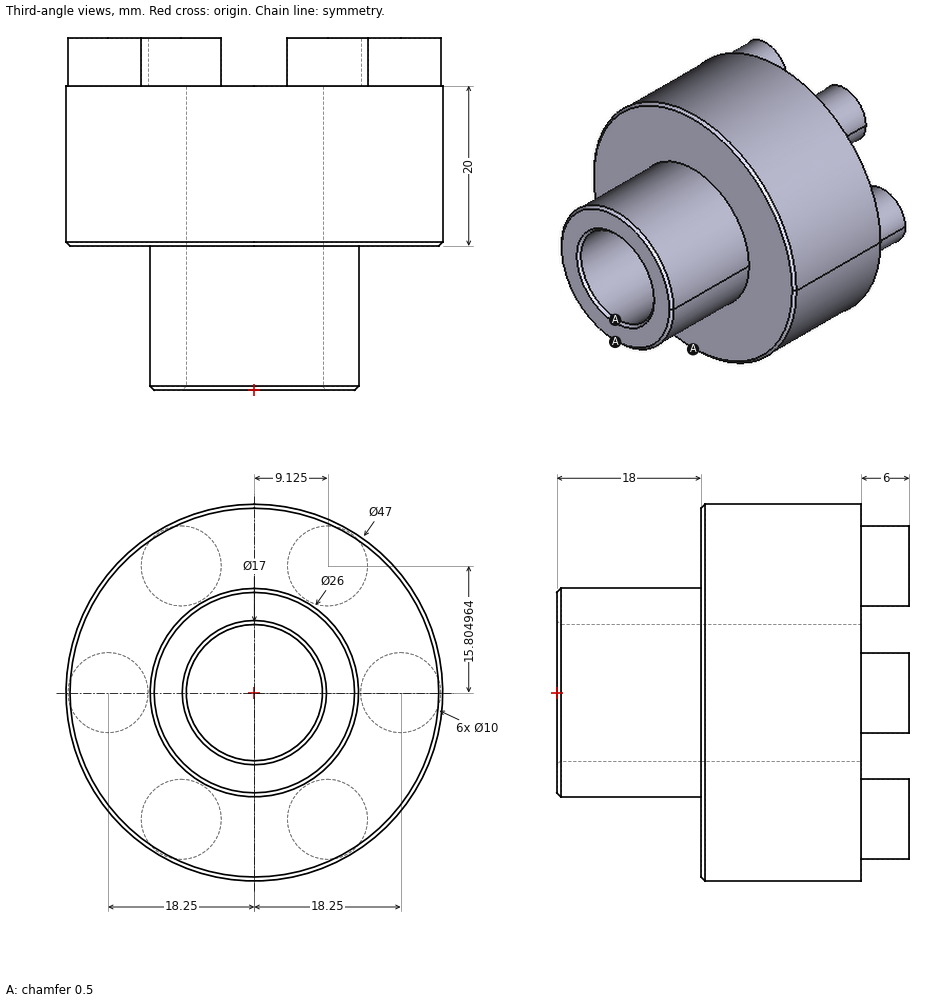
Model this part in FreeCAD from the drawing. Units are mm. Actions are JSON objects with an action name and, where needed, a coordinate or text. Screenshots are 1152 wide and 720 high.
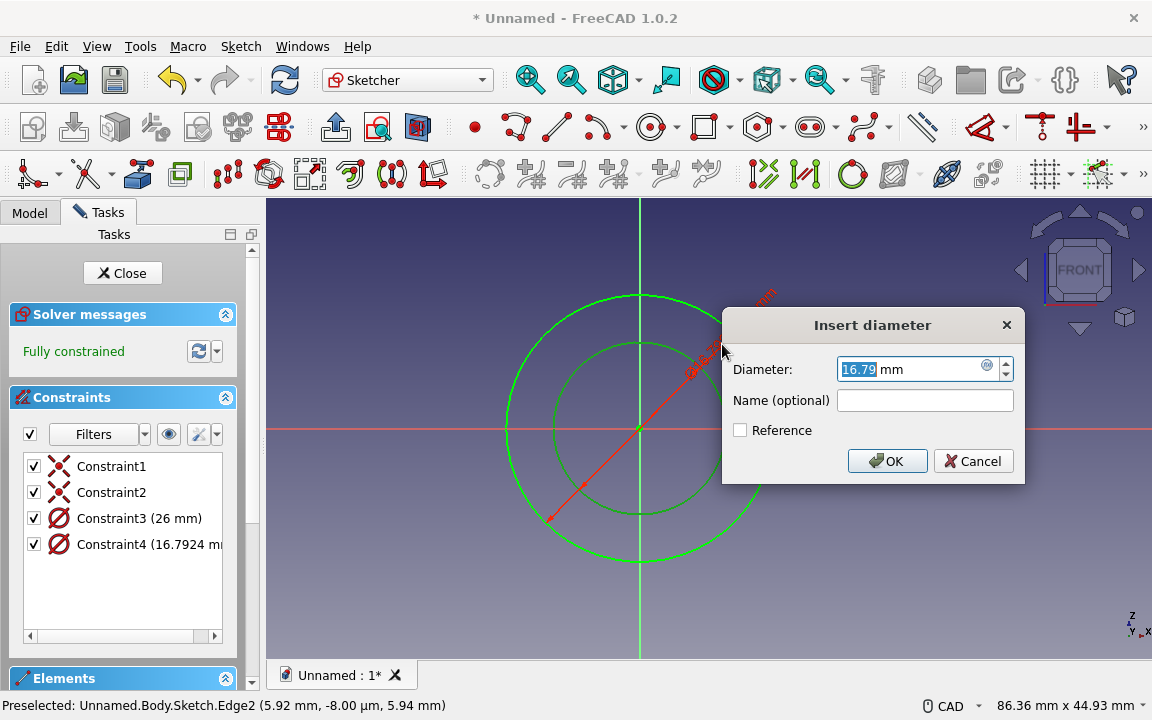
{"action": "type", "text": "17"}
{"action": "key", "text": "Return"}
{"action": "key", "text": "Escape"}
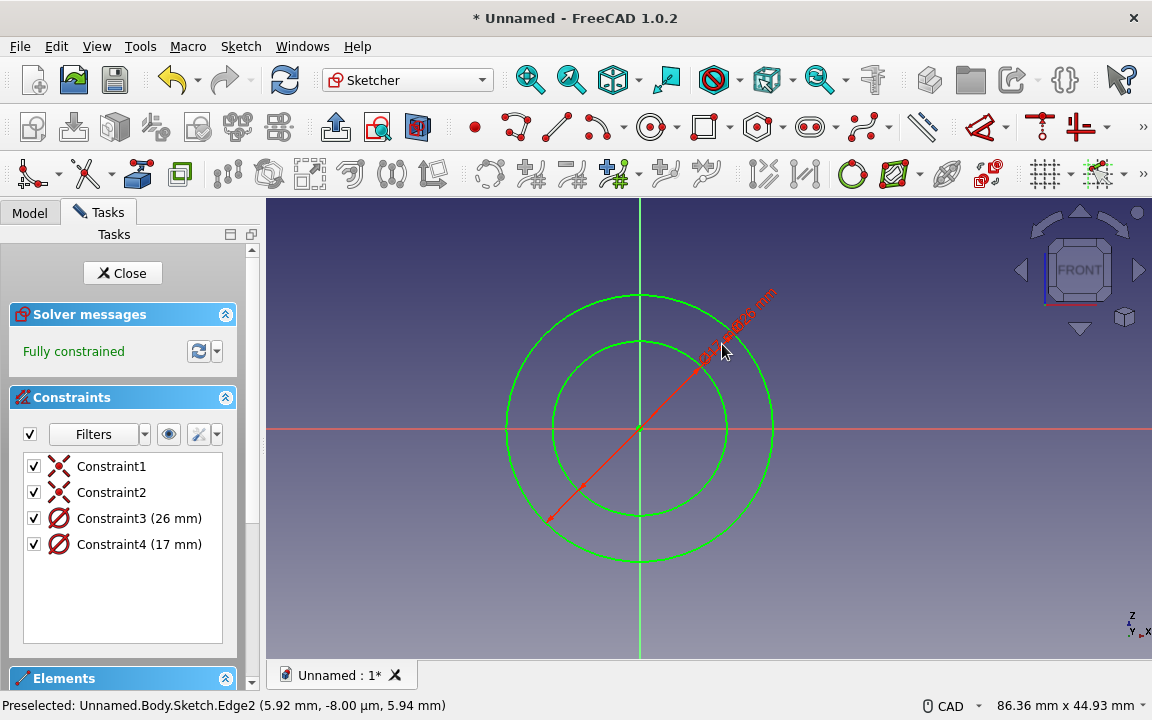
{"action": "left_click", "coordinate": [123, 273]}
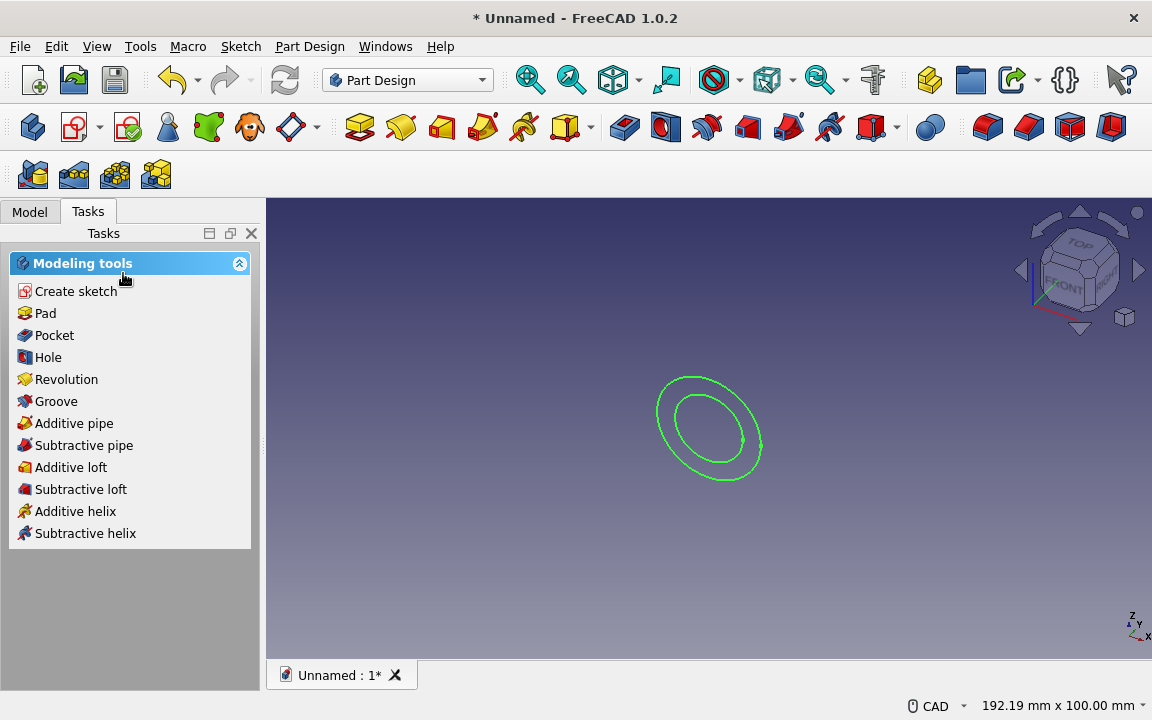
{"action": "left_click", "coordinate": [360, 128]}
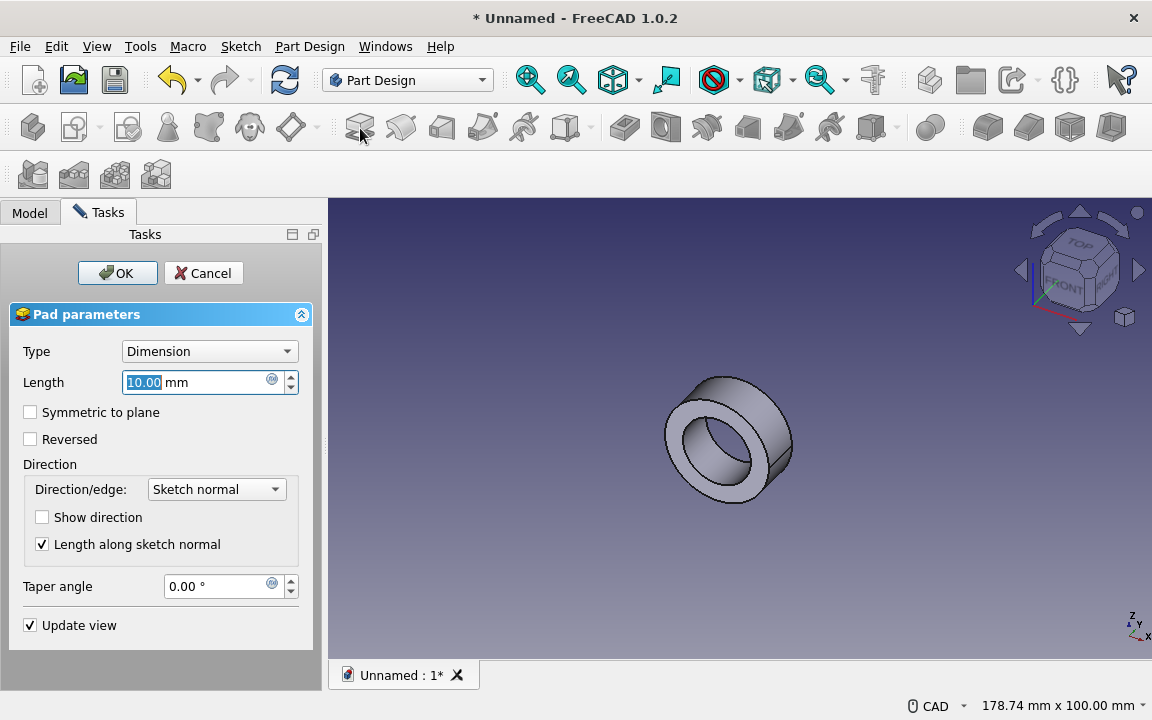
{"action": "type", "text": "18"}
{"action": "key", "text": "Tab"}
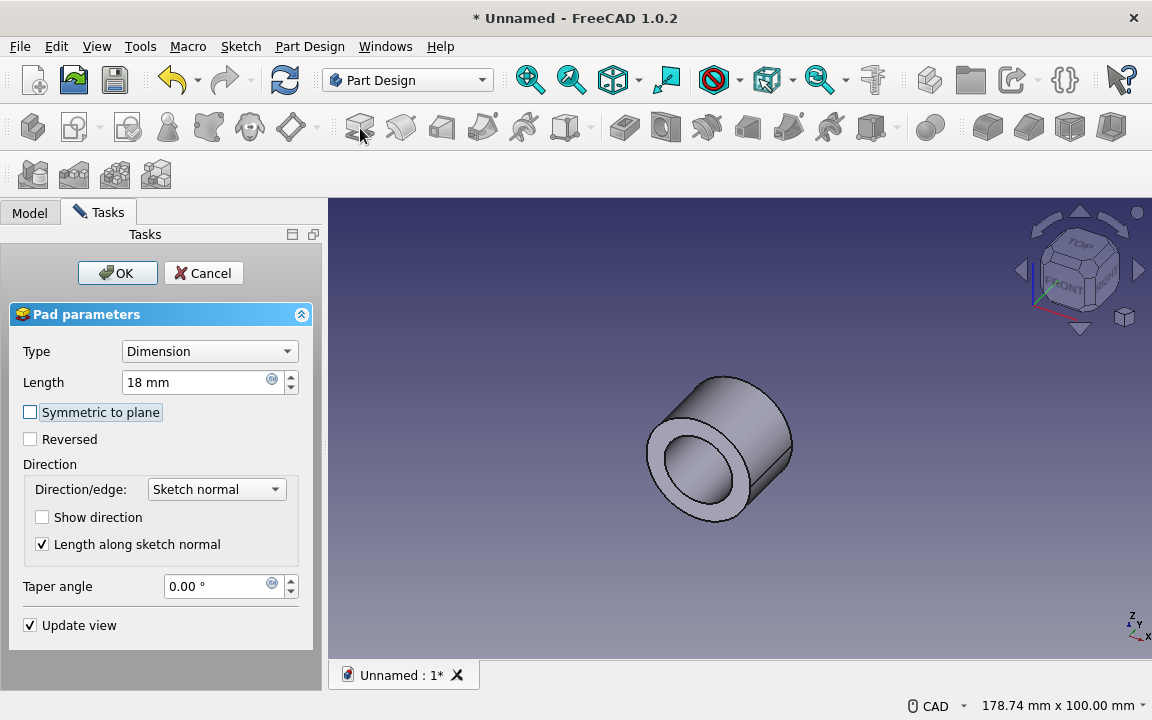
{"action": "left_click", "coordinate": [31, 439]}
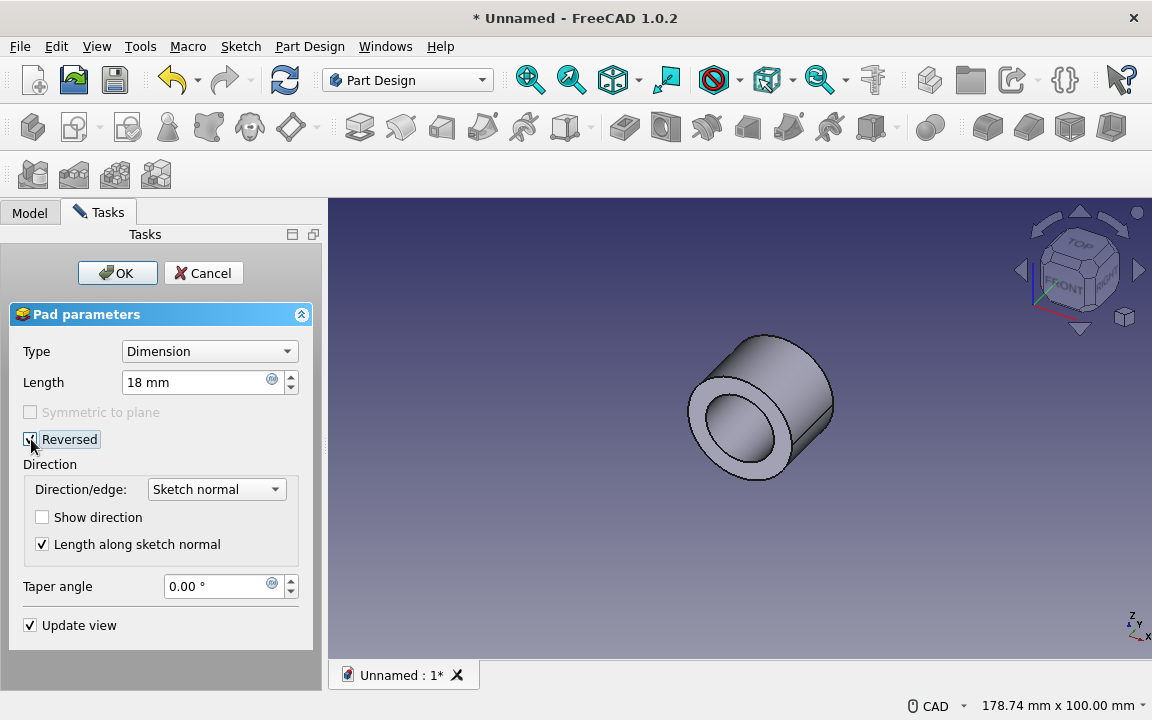
{"action": "left_click", "coordinate": [118, 273]}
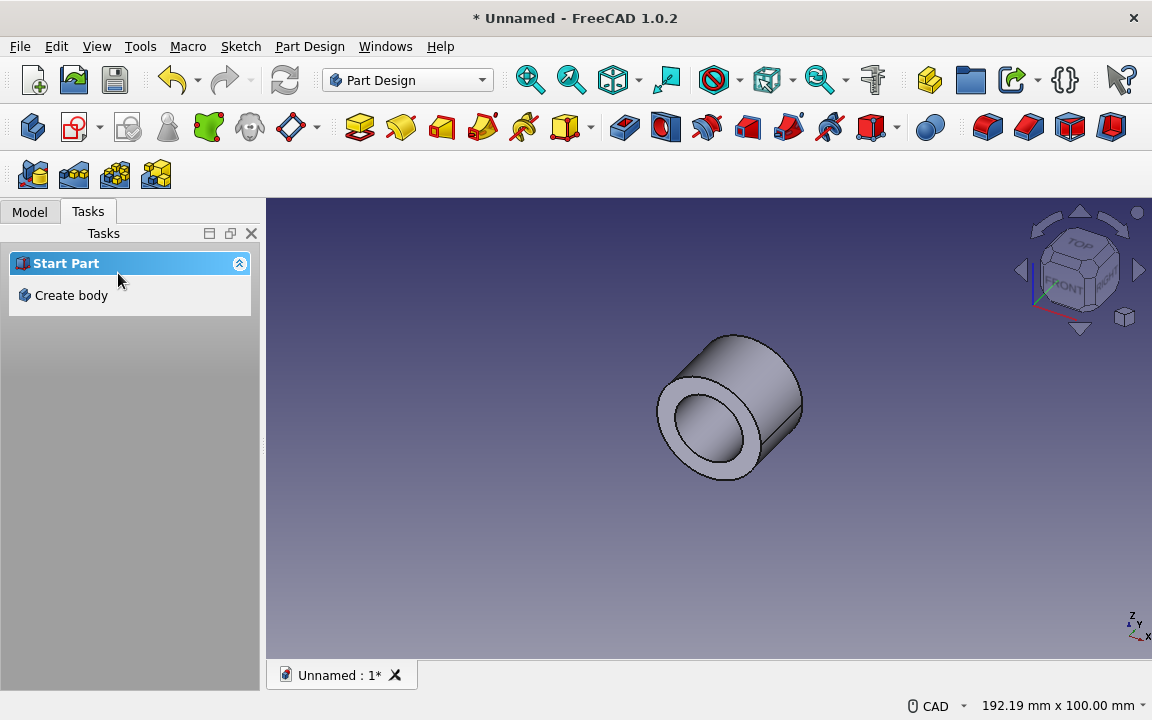
{"action": "left_click", "coordinate": [531, 80]}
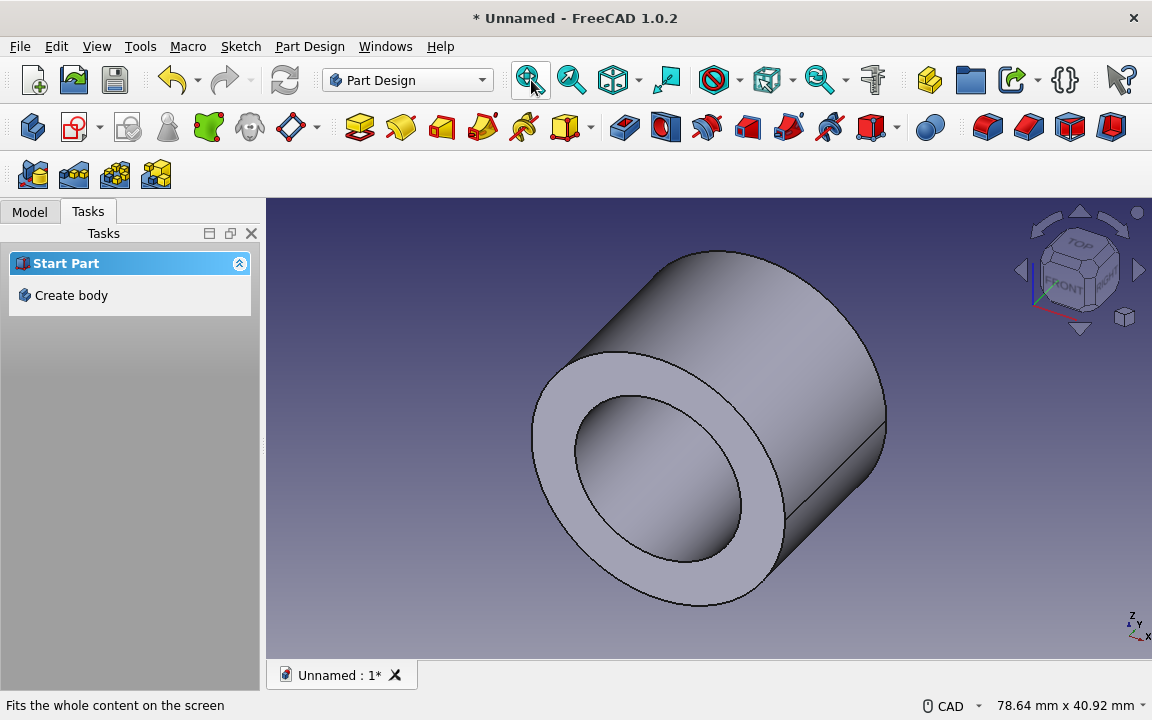
{"action": "key", "text": "4"}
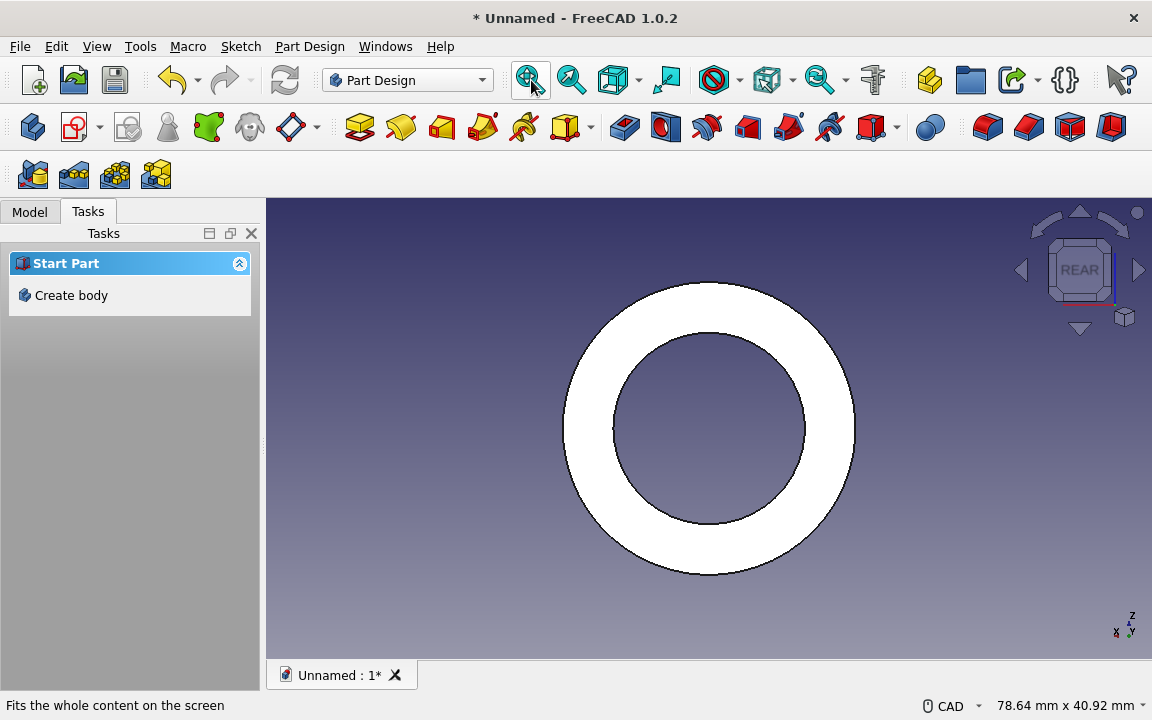
{"action": "left_click", "coordinate": [793, 344]}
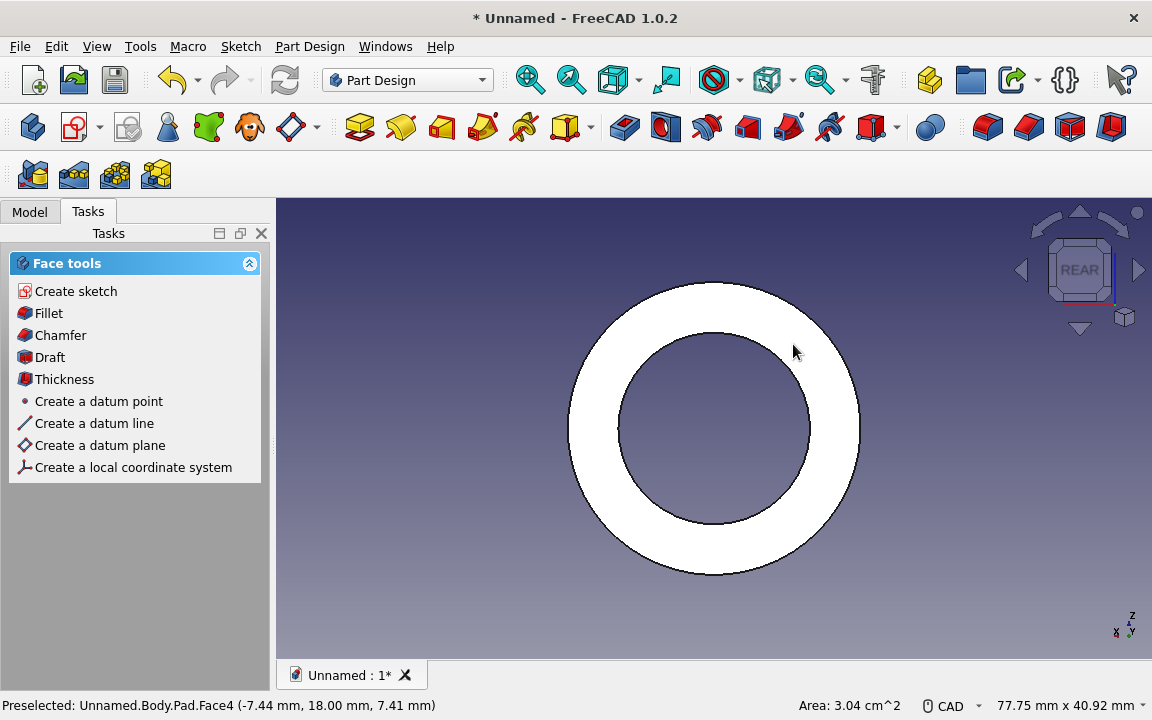
{"action": "left_click", "coordinate": [74, 128]}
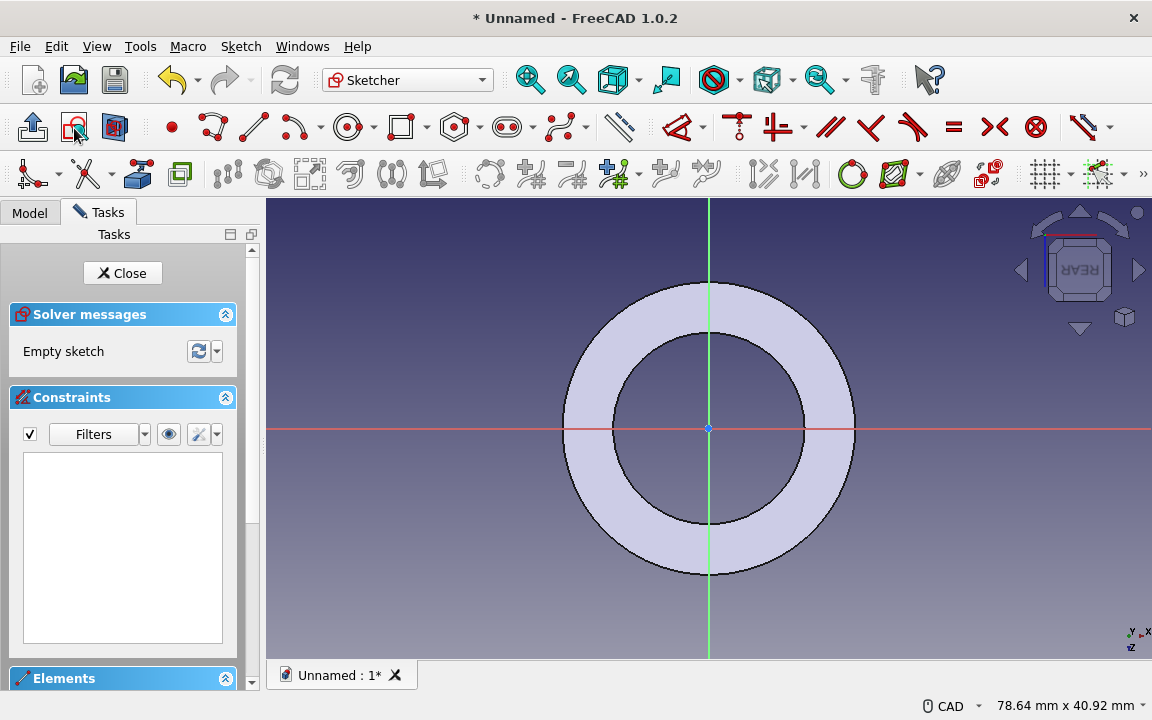
{"action": "scroll", "coordinate": [557, 428], "scroll_direction": "down", "scroll_amount": 3}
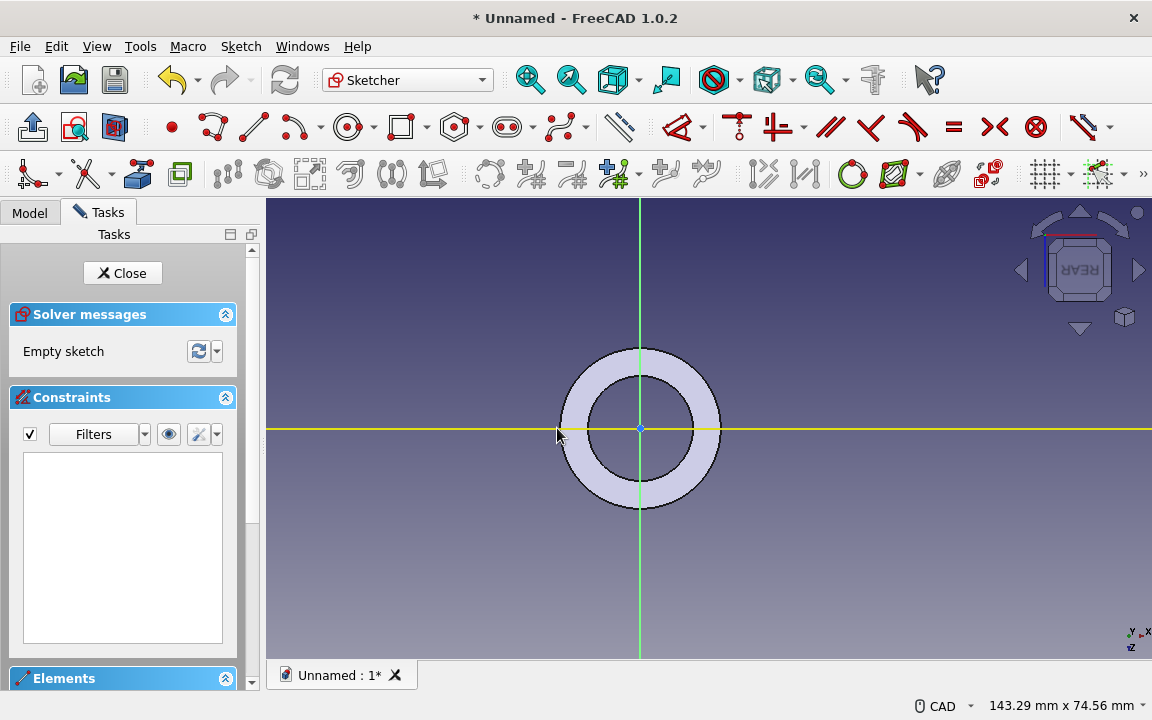
{"action": "left_click", "coordinate": [348, 128]}